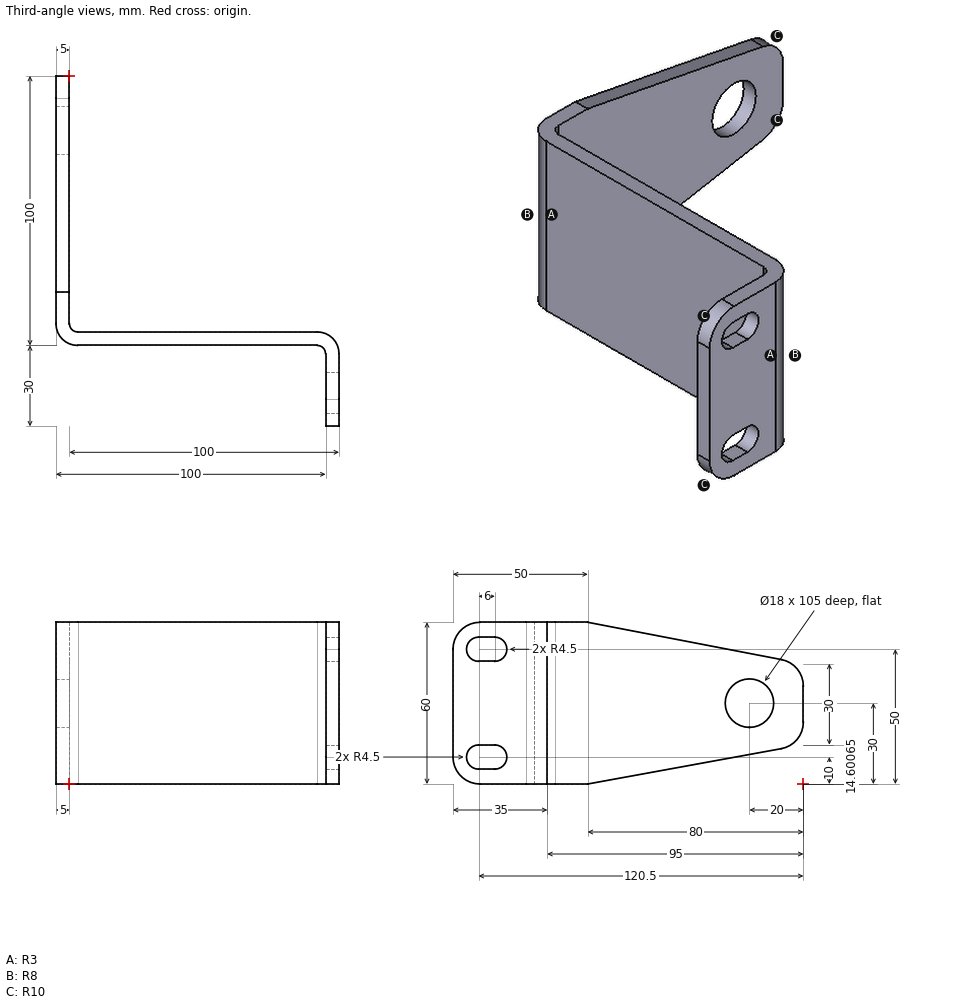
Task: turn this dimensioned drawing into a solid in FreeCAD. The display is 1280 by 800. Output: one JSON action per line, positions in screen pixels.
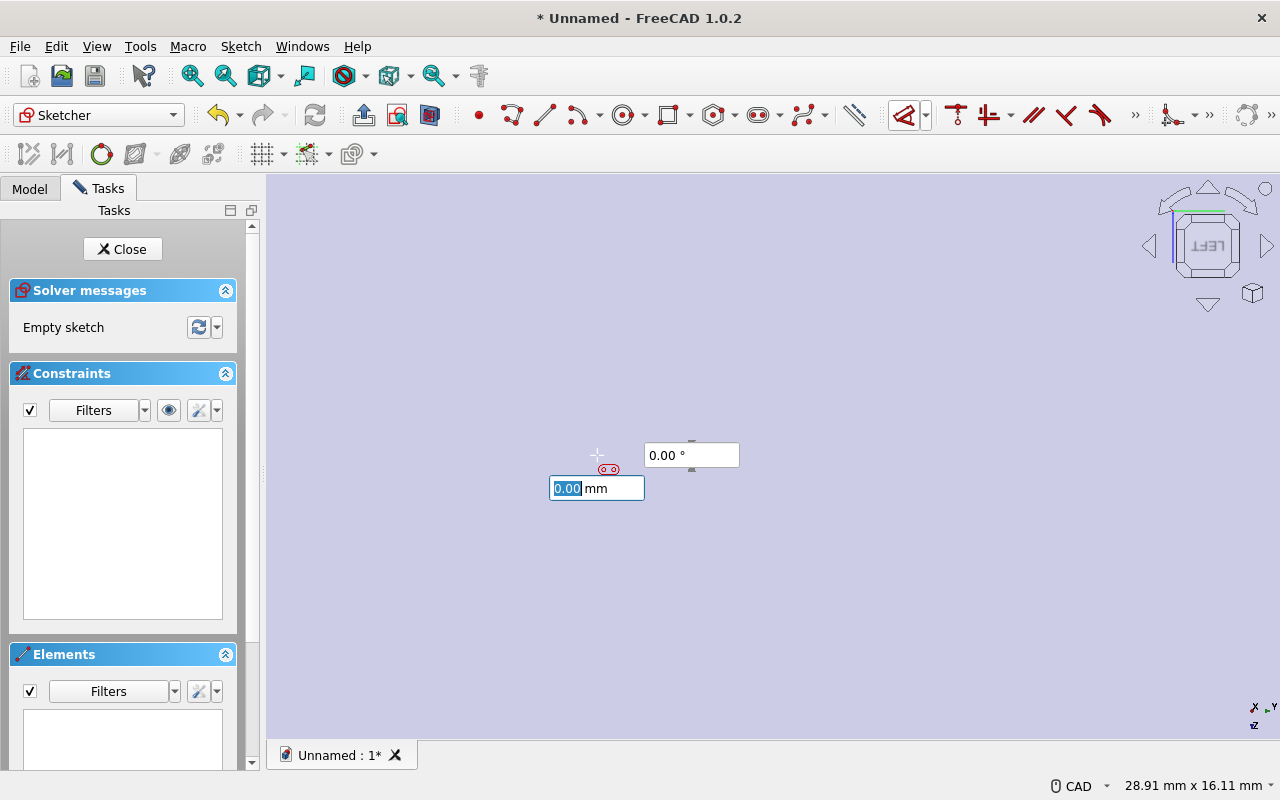
{"action": "left_click", "coordinate": [808, 455]}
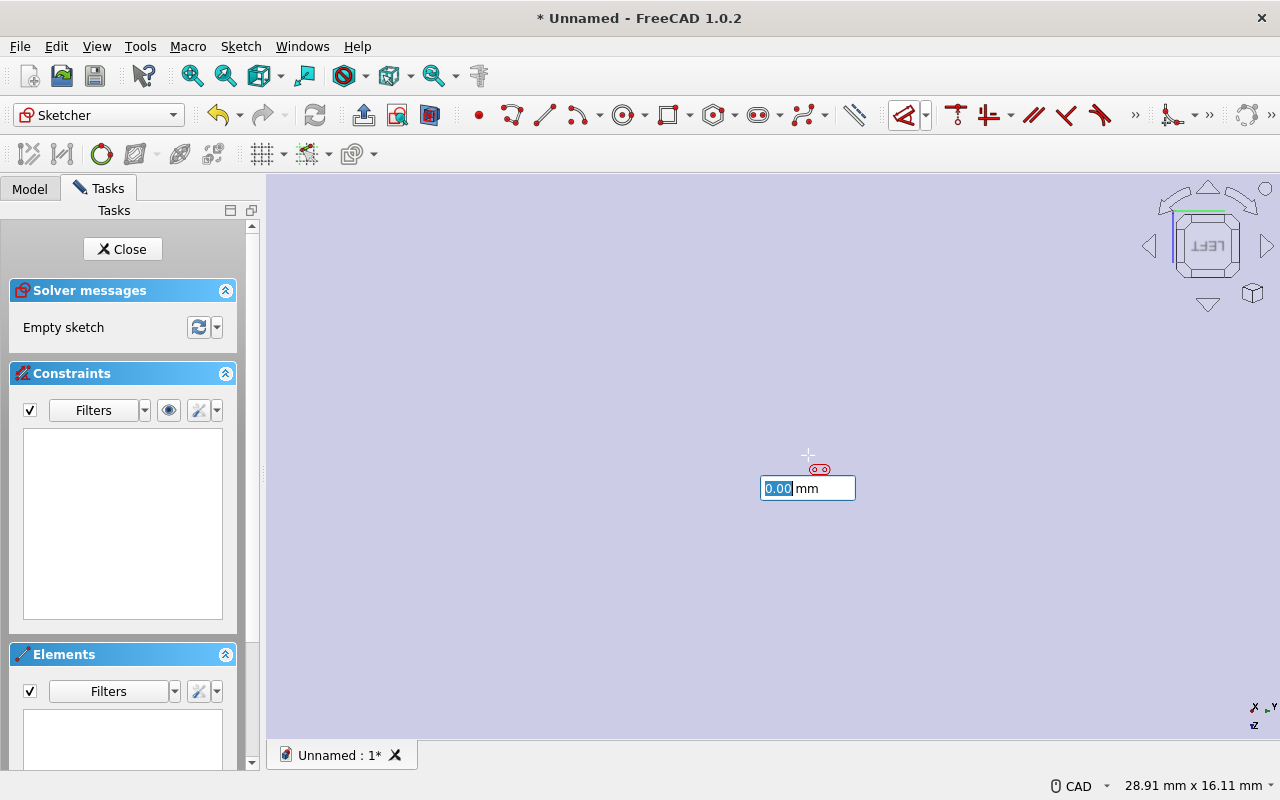
{"action": "left_click", "coordinate": [702, 613]}
{"action": "key", "text": "Escape"}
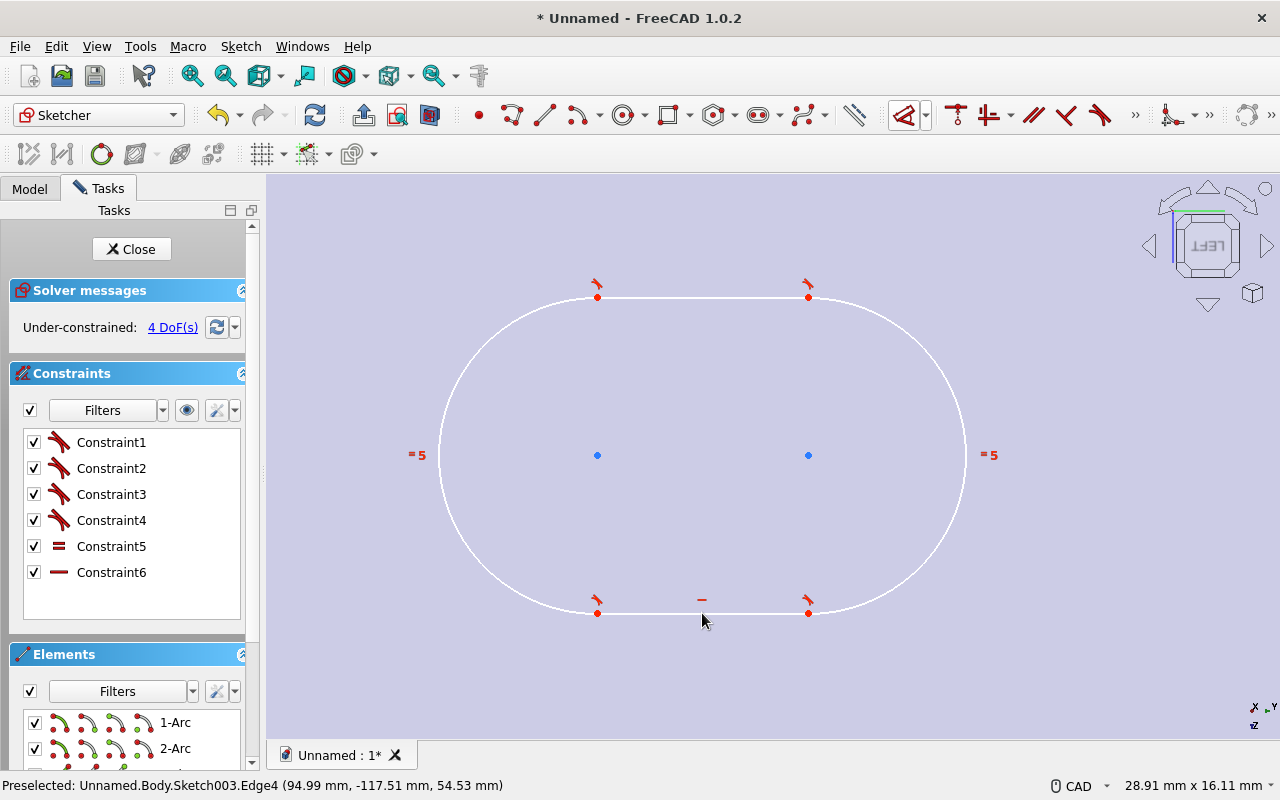
{"action": "left_click", "coordinate": [469, 363]}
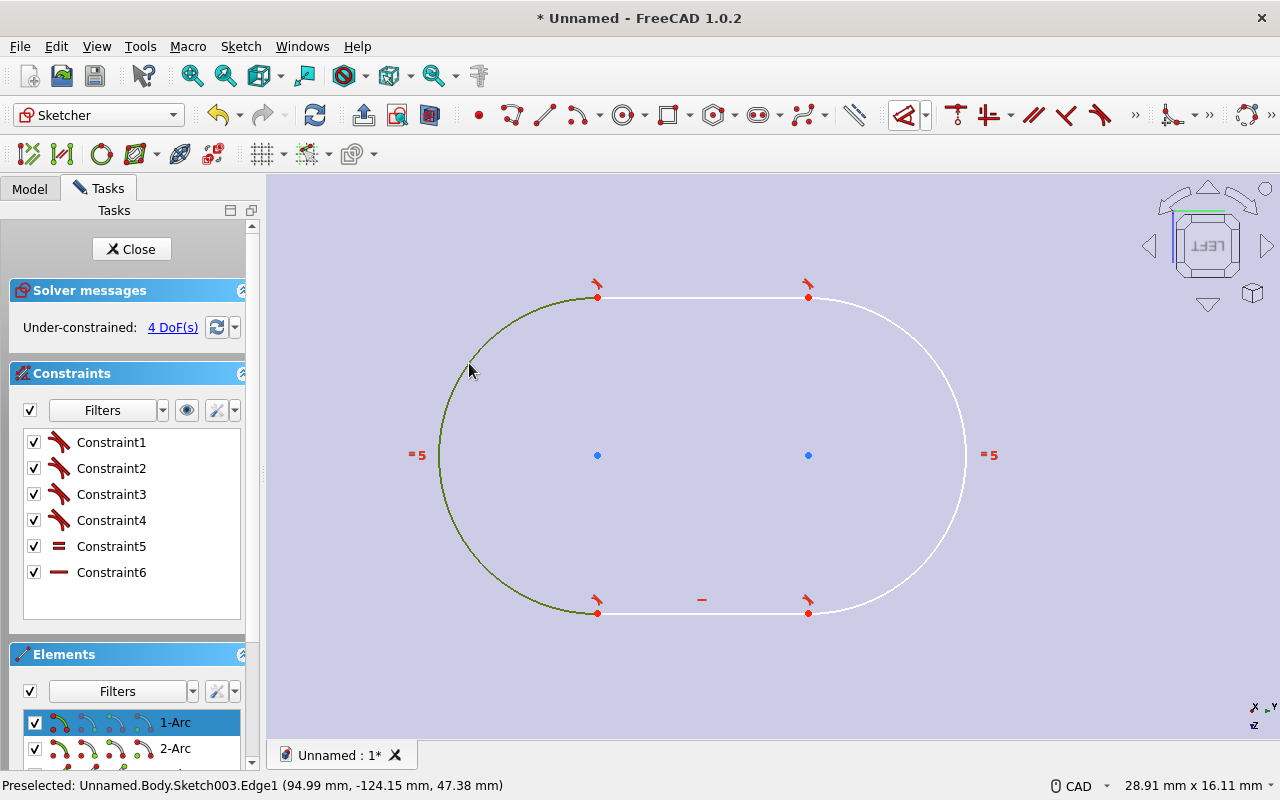
{"action": "left_click", "coordinate": [926, 116]}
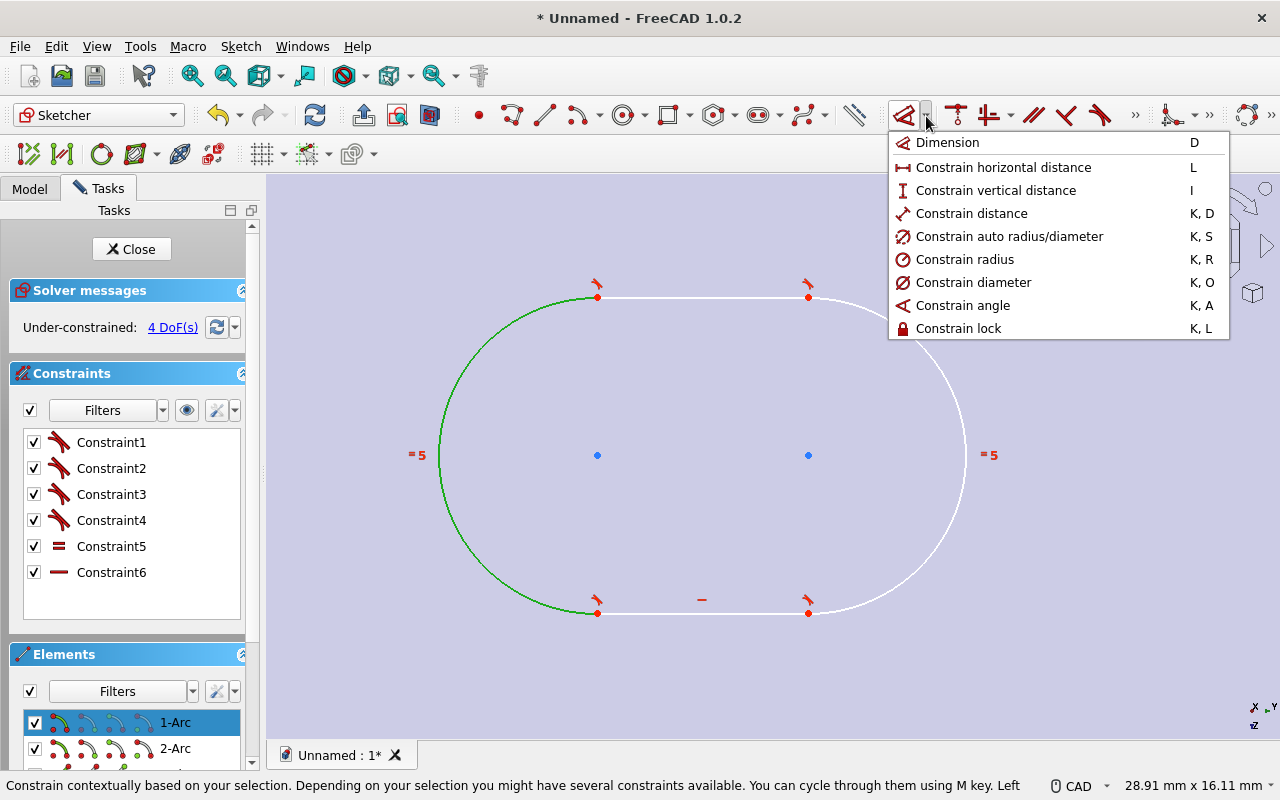
{"action": "left_click", "coordinate": [1059, 260]}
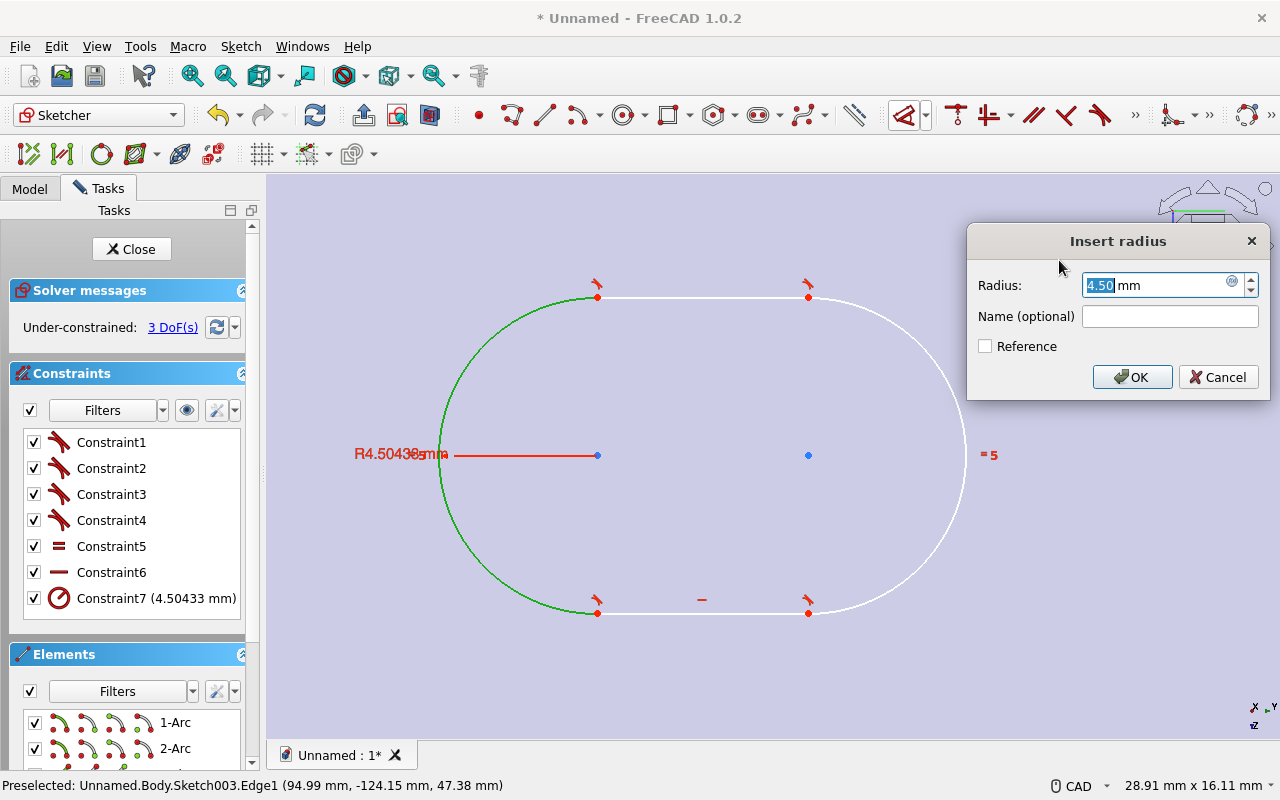
{"action": "type", "text": "4.5"}
{"action": "key", "text": "Return"}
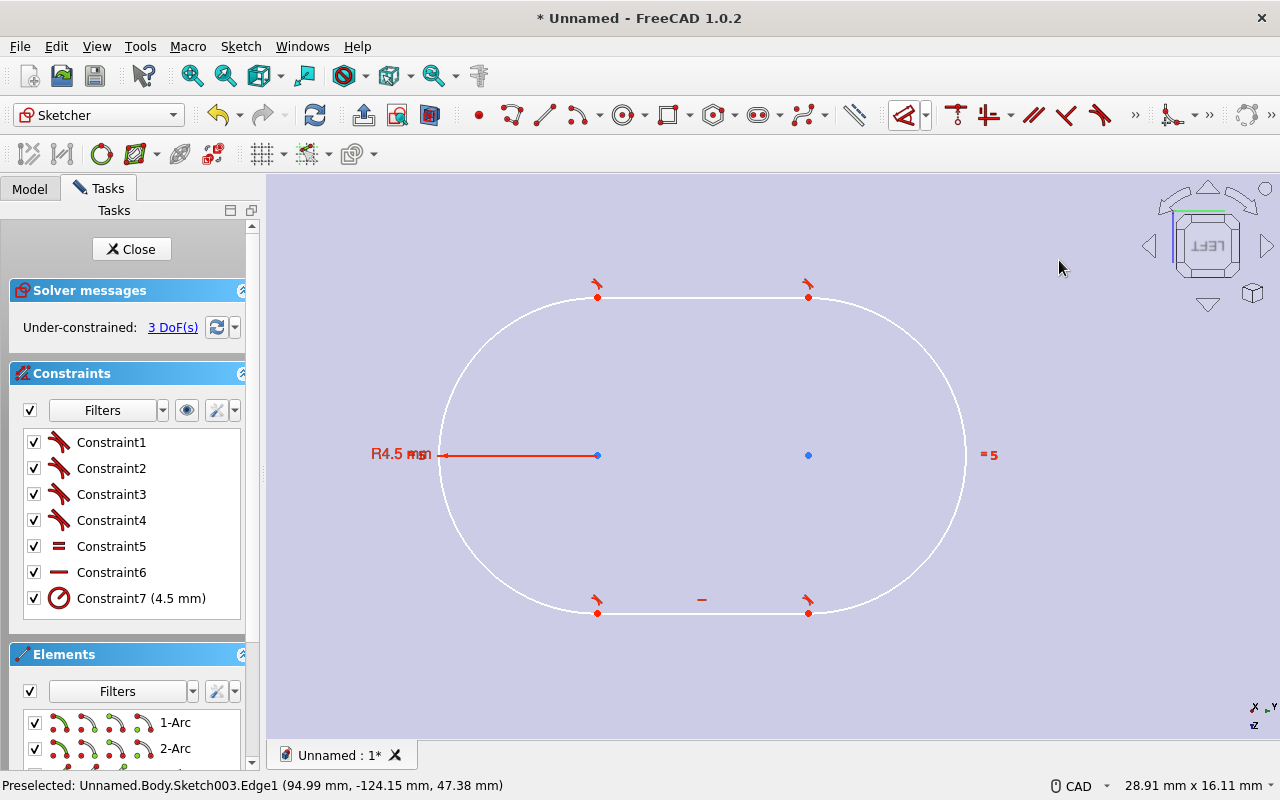
{"action": "left_click", "coordinate": [660, 298]}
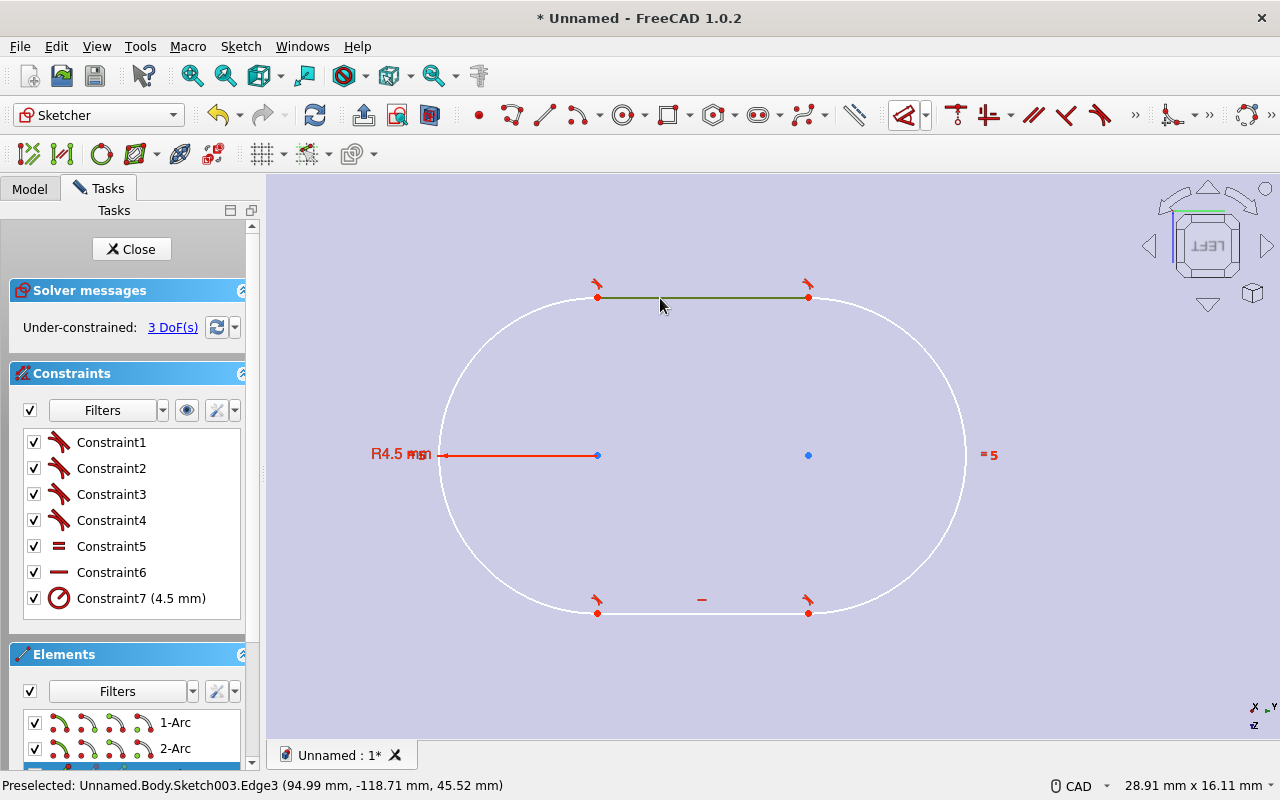
{"action": "left_click", "coordinate": [926, 116]}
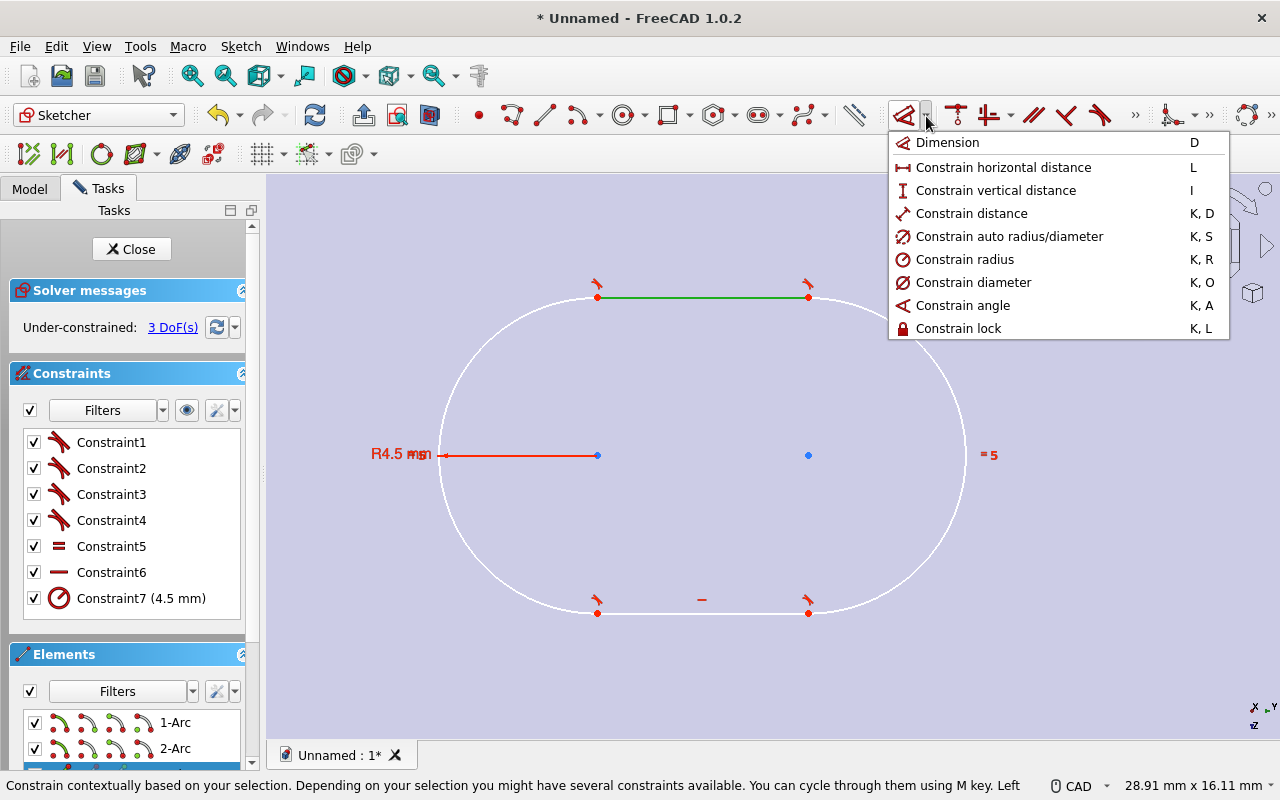
{"action": "left_click", "coordinate": [1059, 168]}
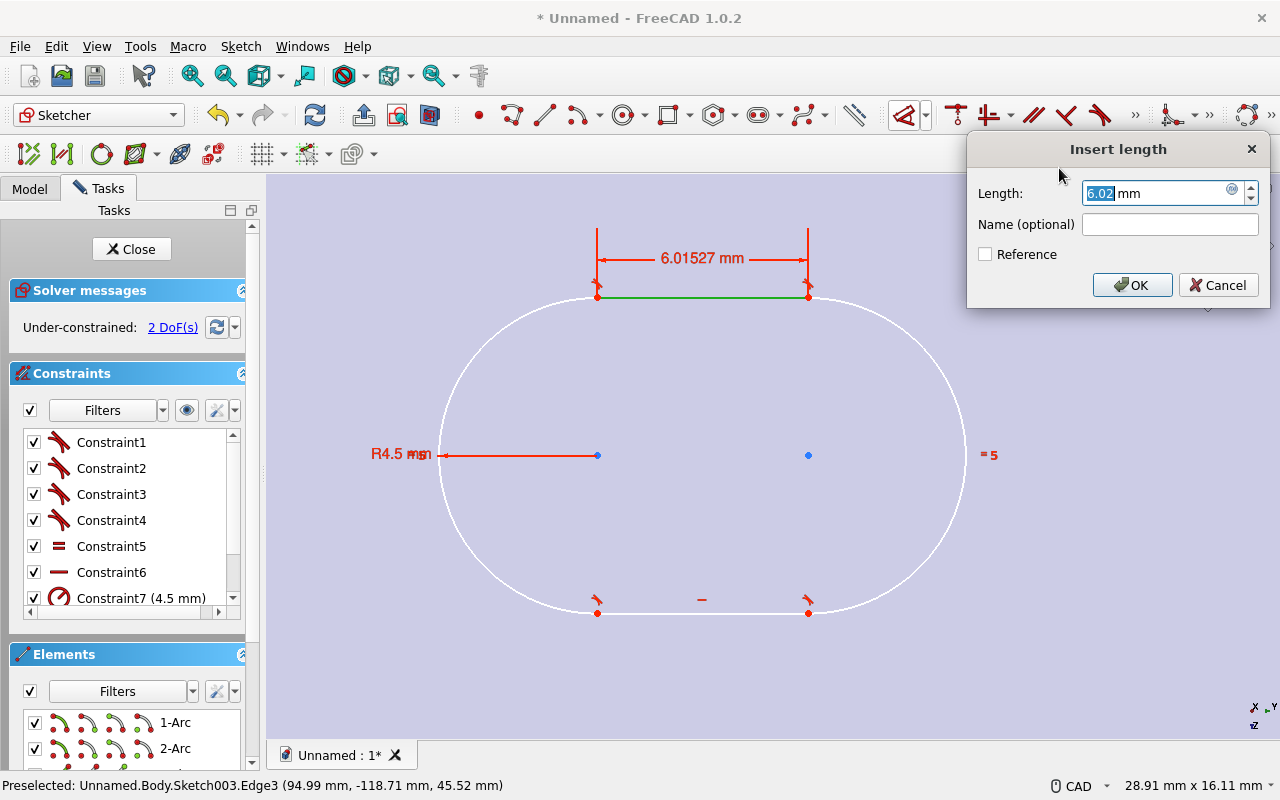
{"action": "type", "text": "6"}
{"action": "key", "text": "Return"}